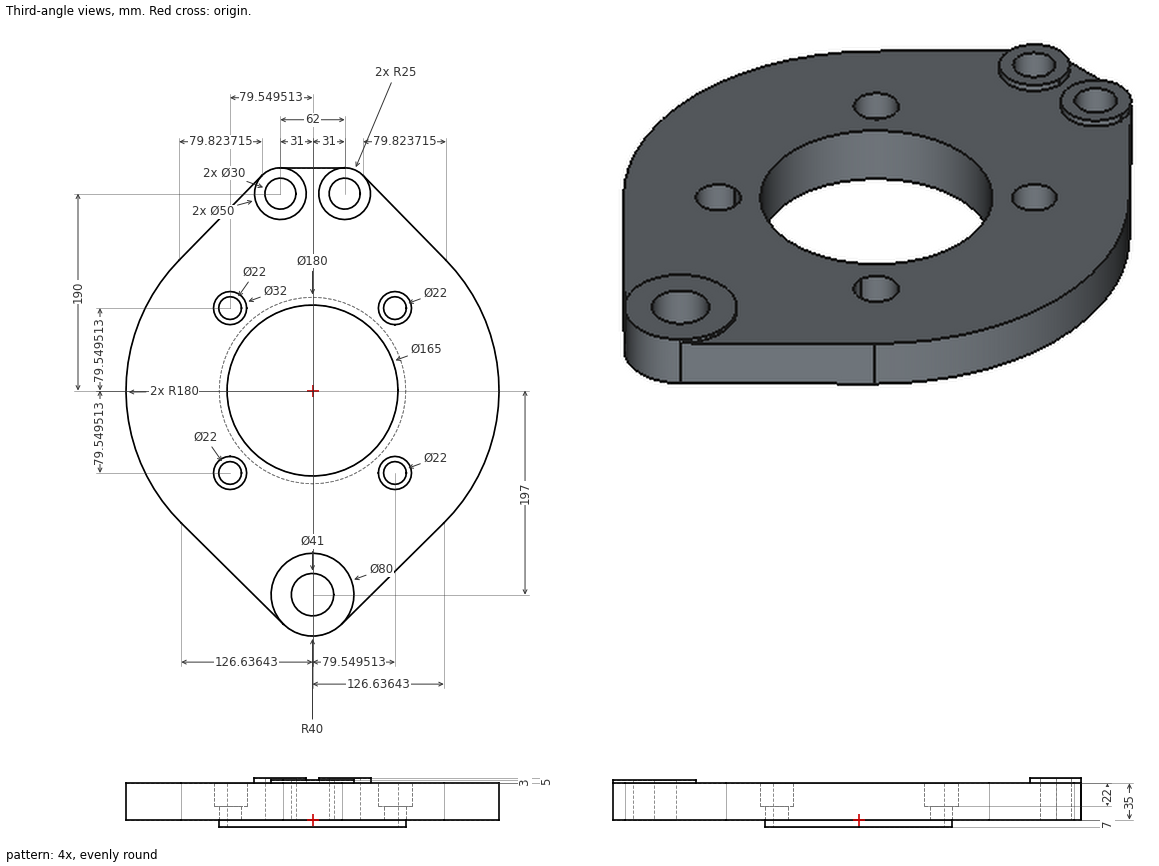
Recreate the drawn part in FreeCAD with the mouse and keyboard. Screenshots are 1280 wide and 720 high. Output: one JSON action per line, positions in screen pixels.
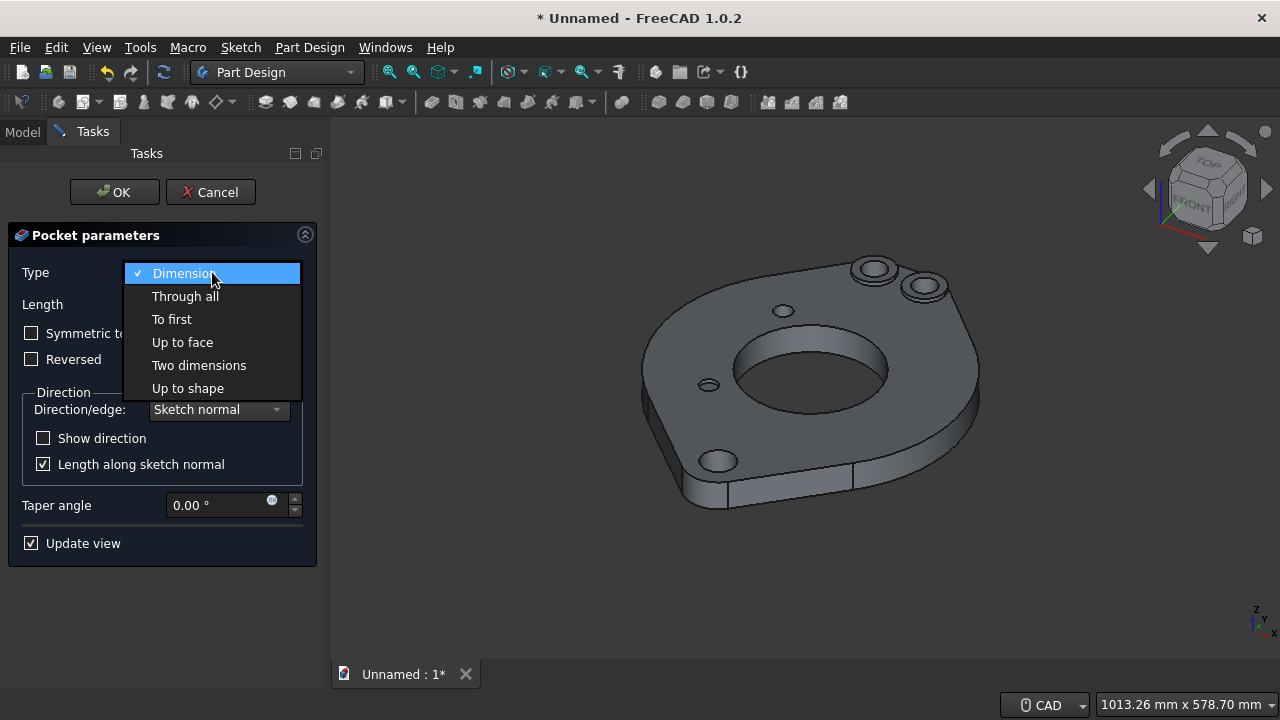
{"action": "left_click", "coordinate": [212, 320]}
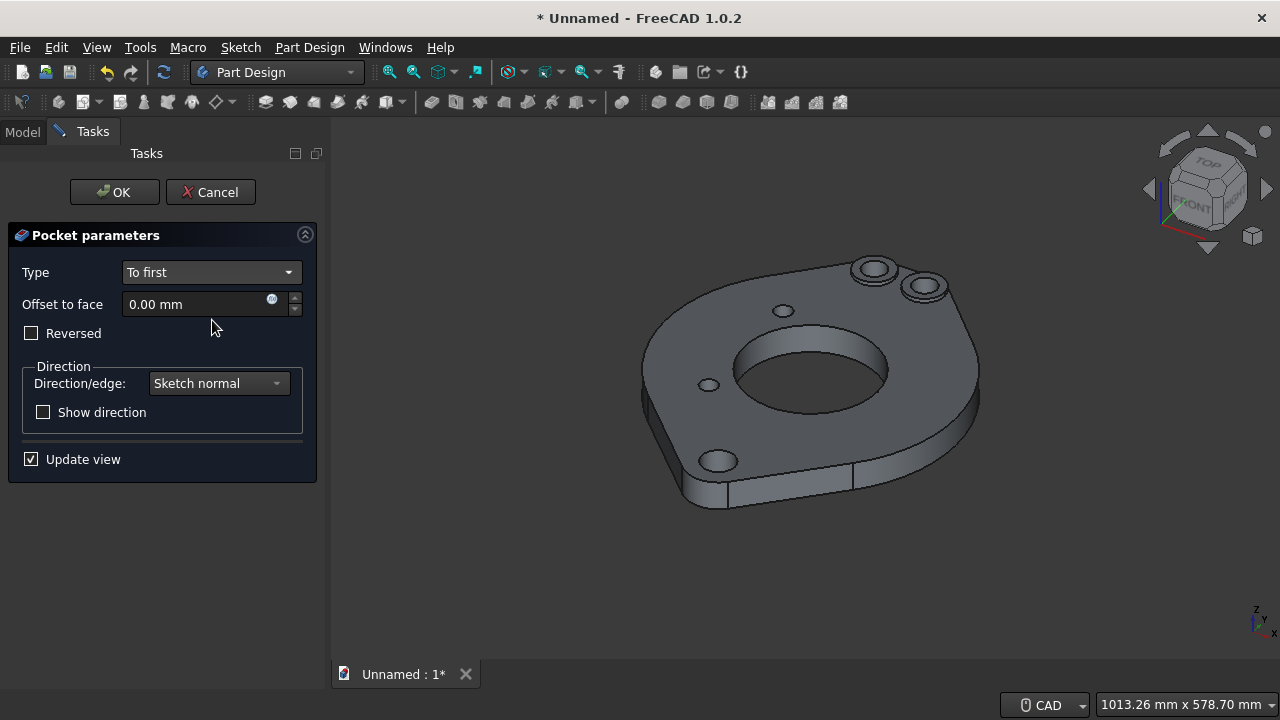
{"action": "left_click", "coordinate": [115, 192]}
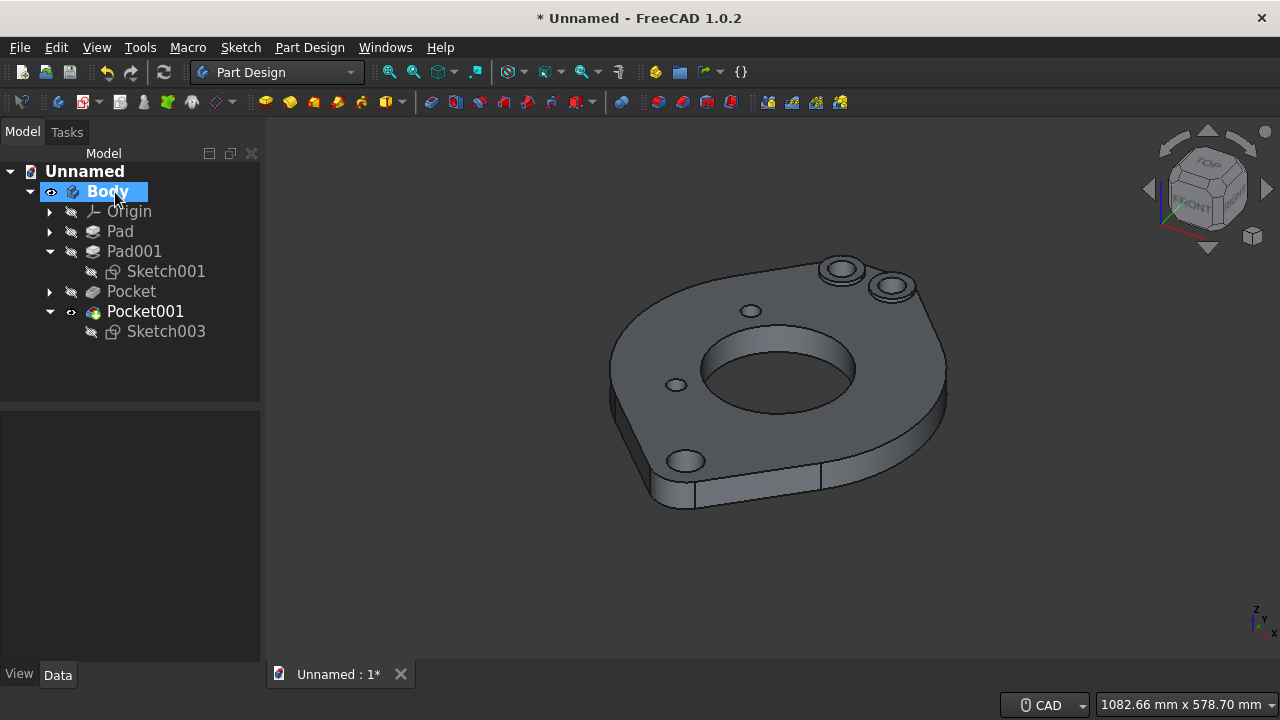
{"action": "left_click", "coordinate": [875, 327]}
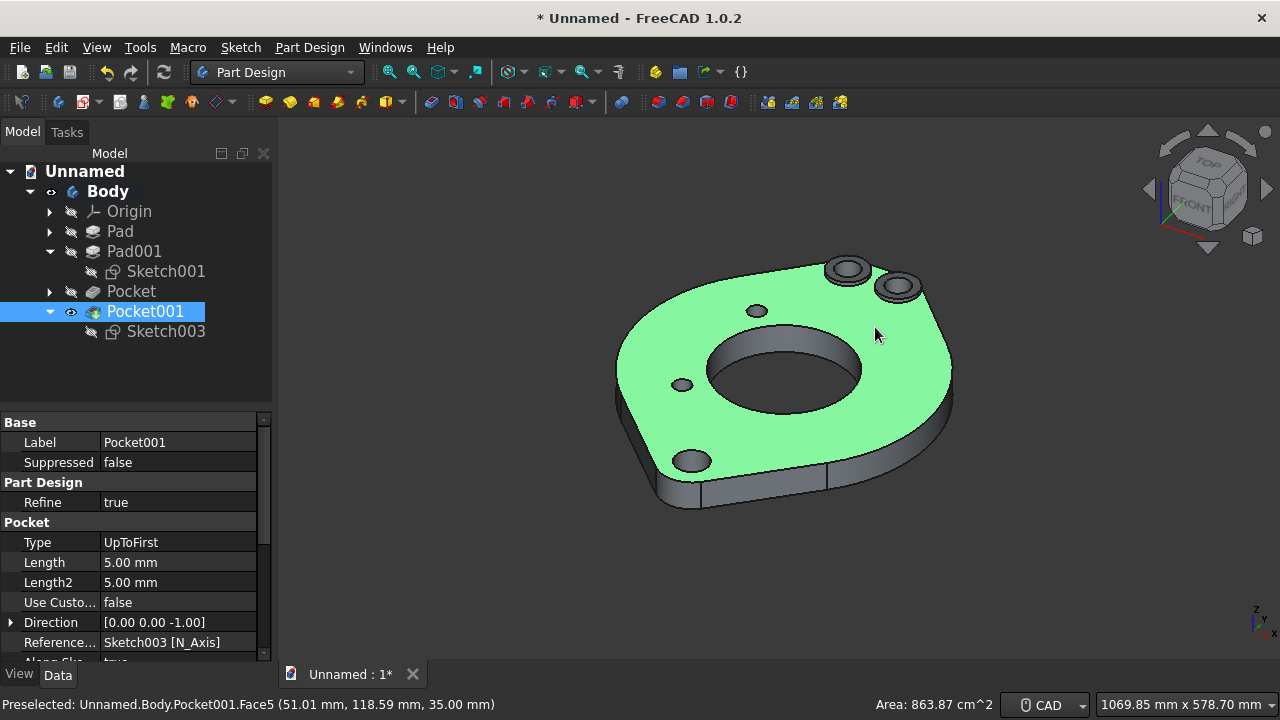
{"action": "left_click", "coordinate": [84, 102]}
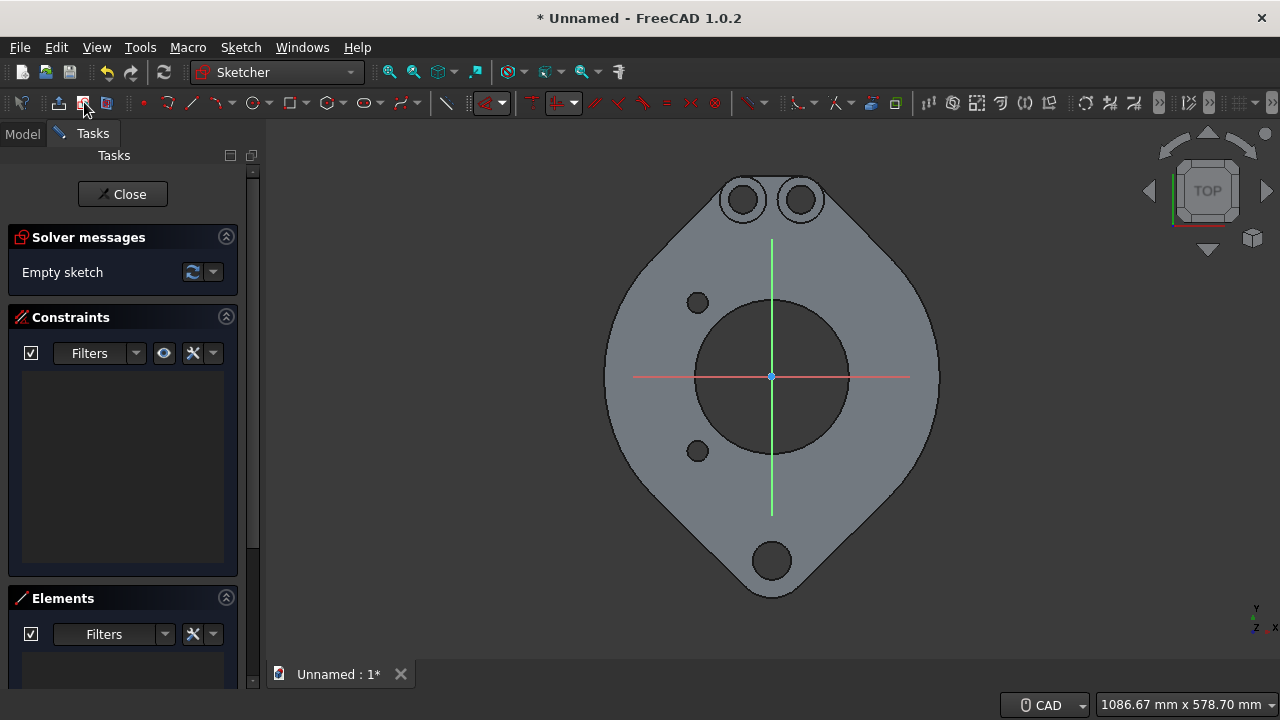
{"action": "left_click", "coordinate": [108, 104]}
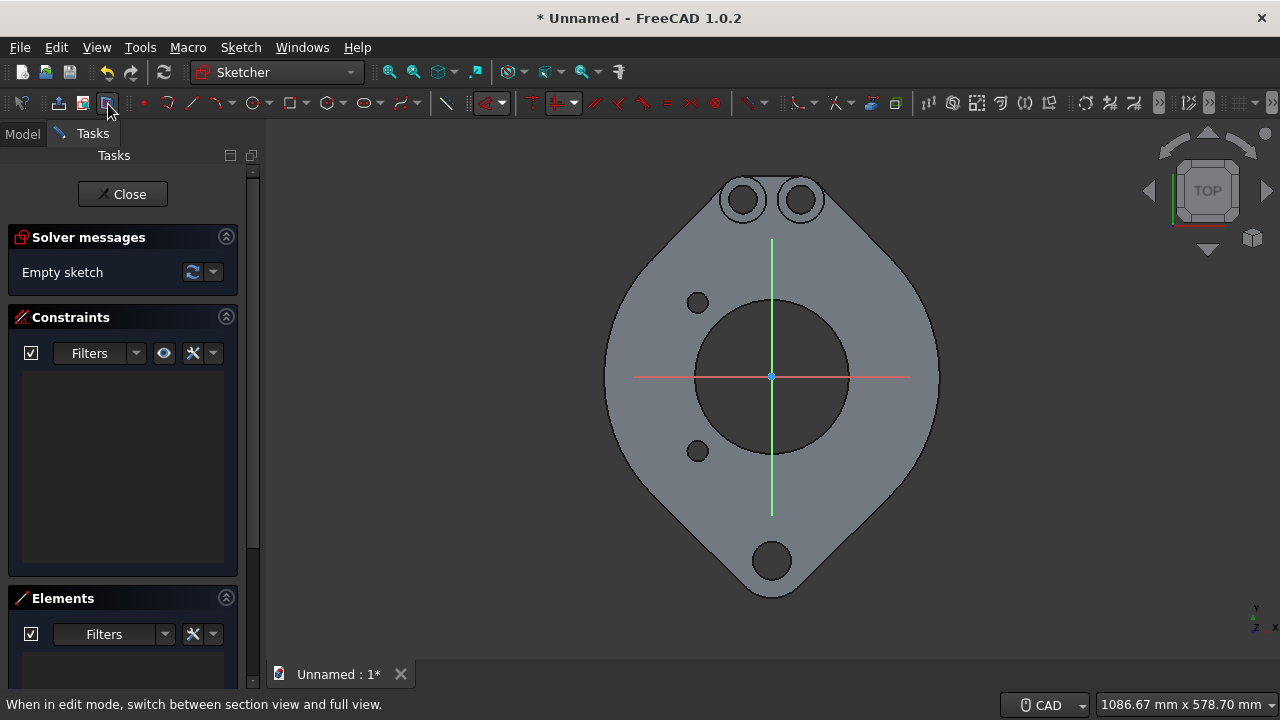
{"action": "scroll", "coordinate": [855, 455], "scroll_direction": "up", "scroll_amount": 14}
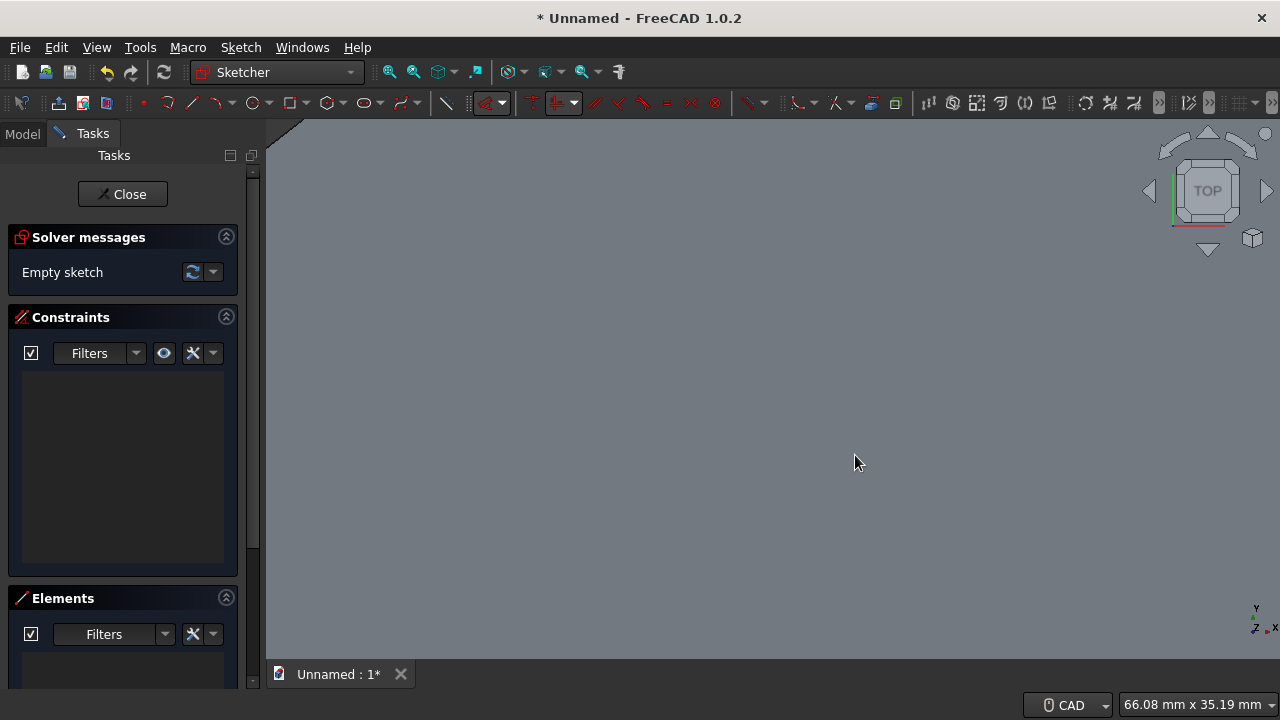
{"action": "key", "text": "g c"}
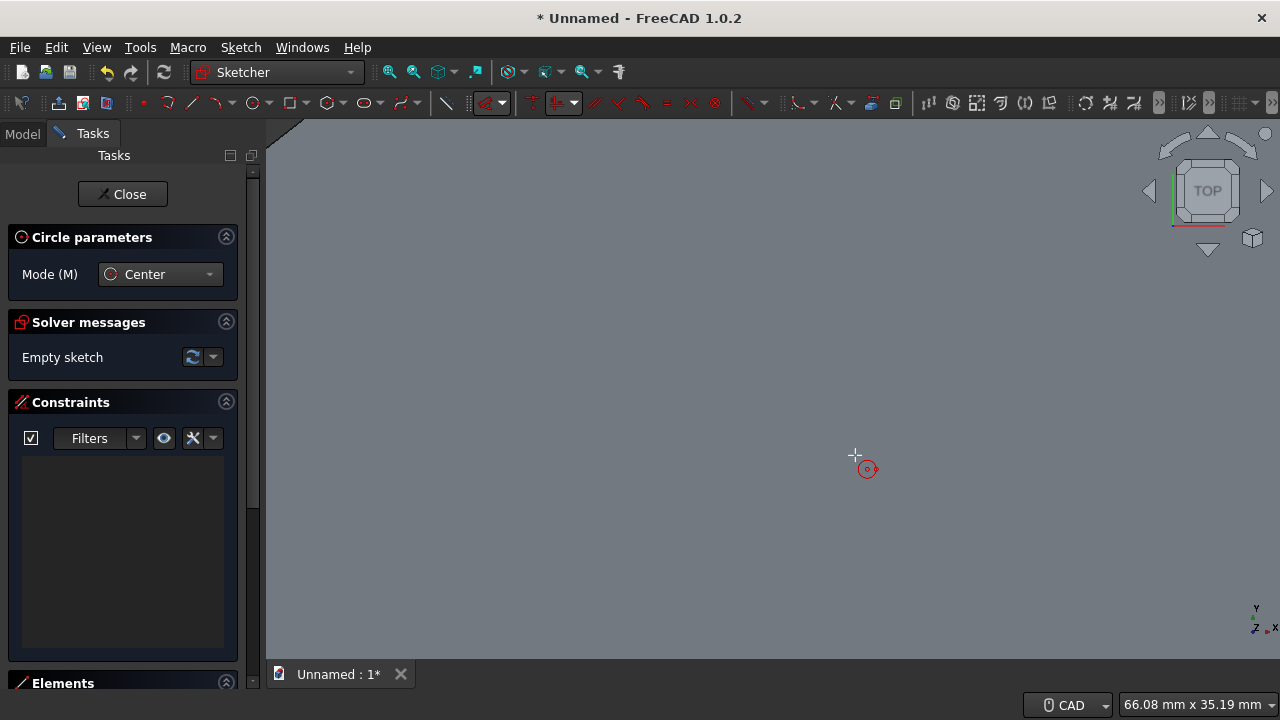
{"action": "left_click", "coordinate": [700, 383]}
{"action": "left_click", "coordinate": [820, 263]}
{"action": "key", "text": "Escape"}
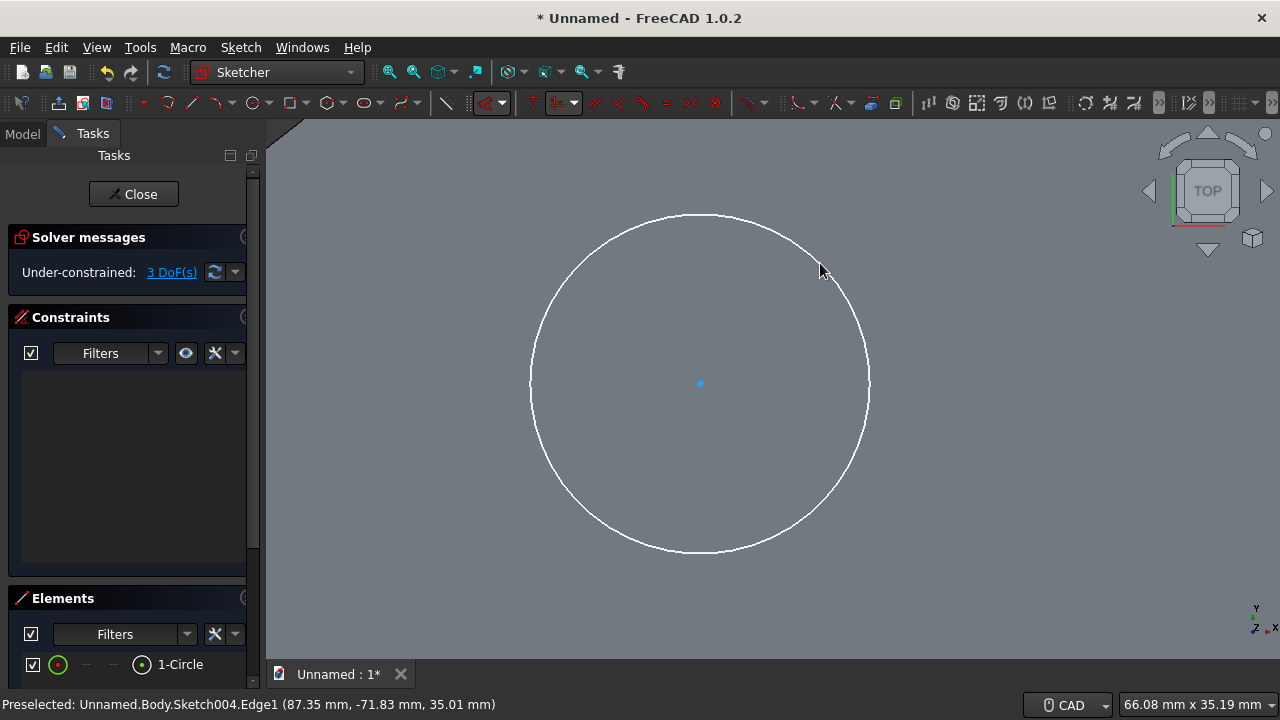
{"action": "left_click", "coordinate": [820, 264]}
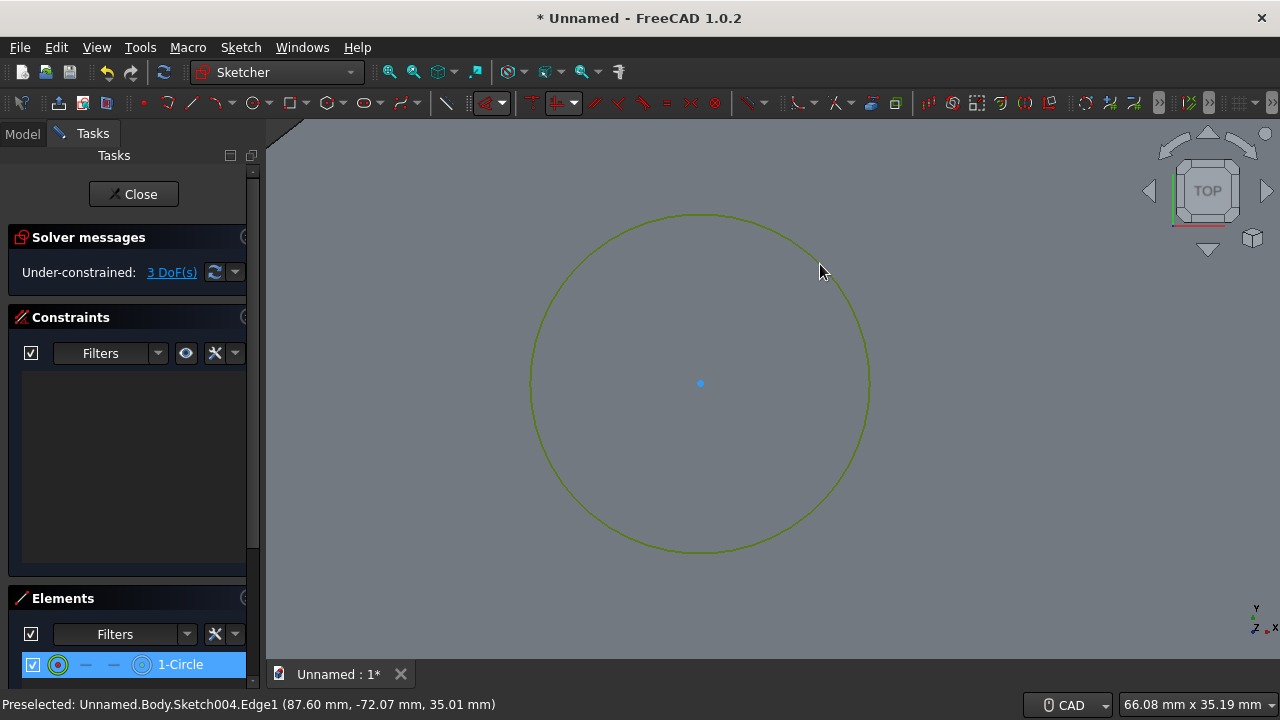
{"action": "key", "text": "k o"}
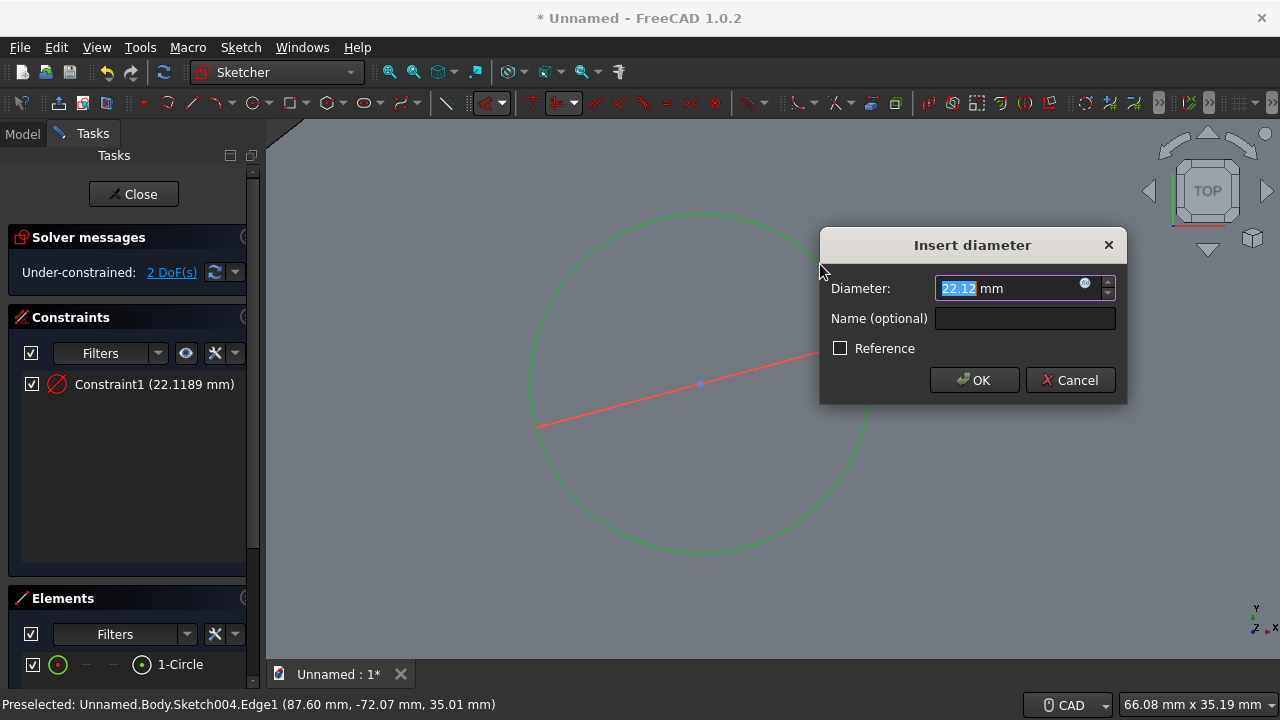
{"action": "type", "text": "22"}
{"action": "key", "text": "Return"}